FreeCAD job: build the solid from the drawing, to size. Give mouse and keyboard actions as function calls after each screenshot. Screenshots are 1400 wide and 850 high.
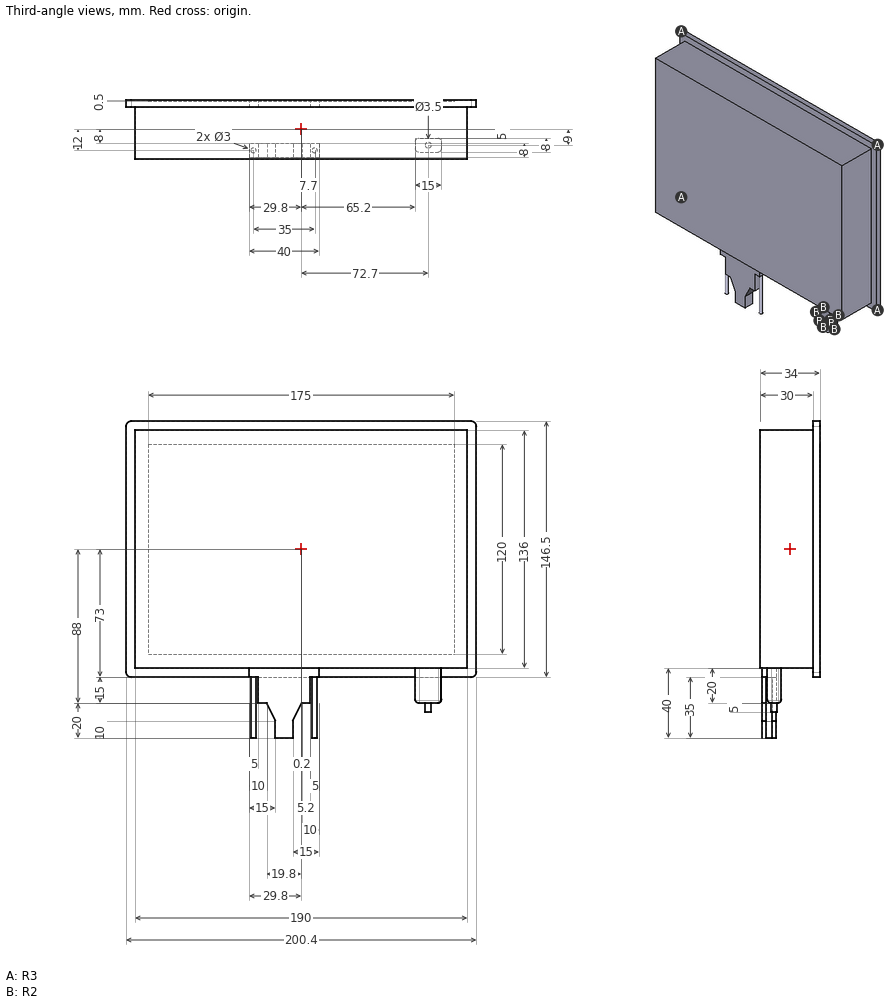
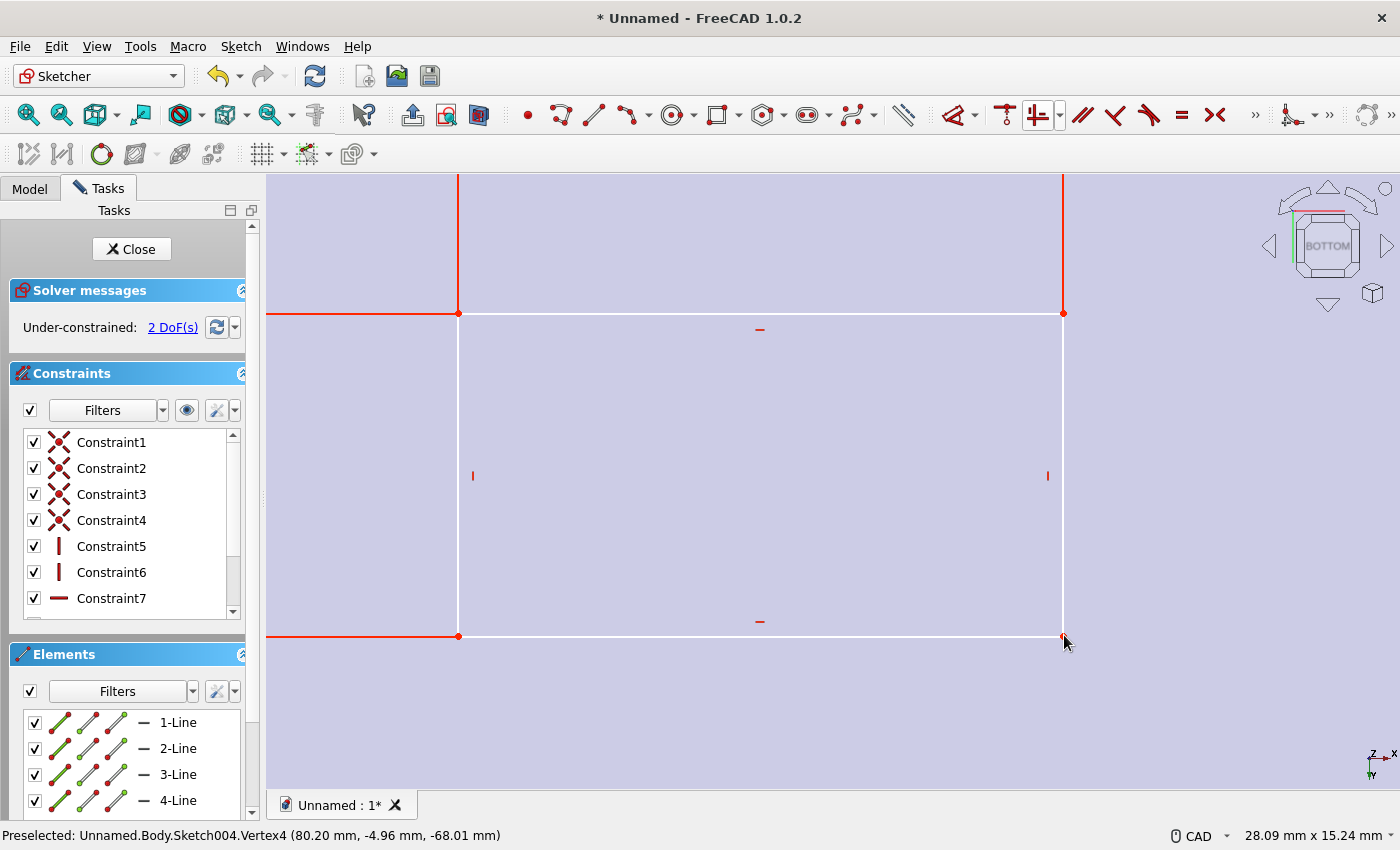
click(952, 116)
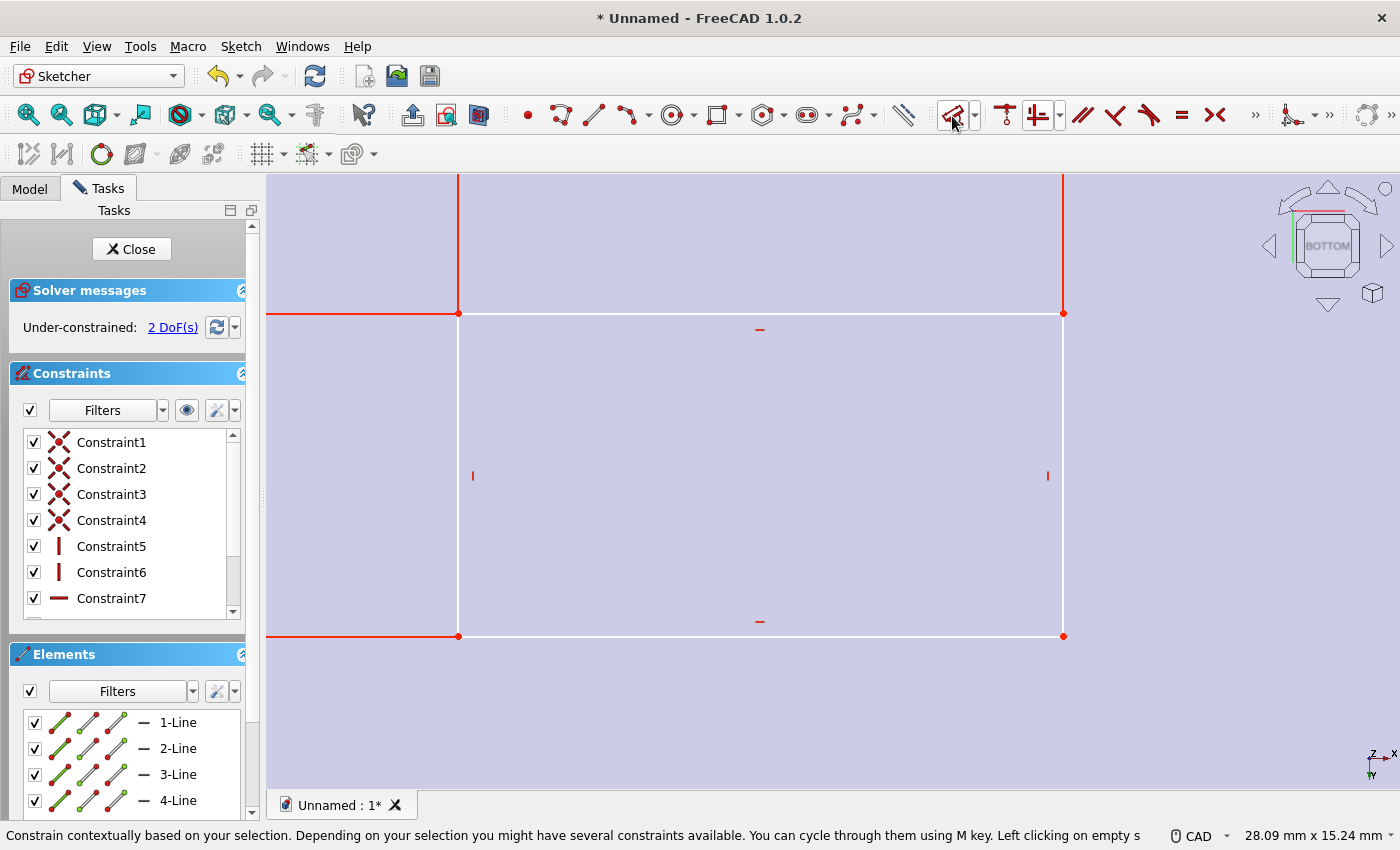
click(458, 637)
click(492, 699)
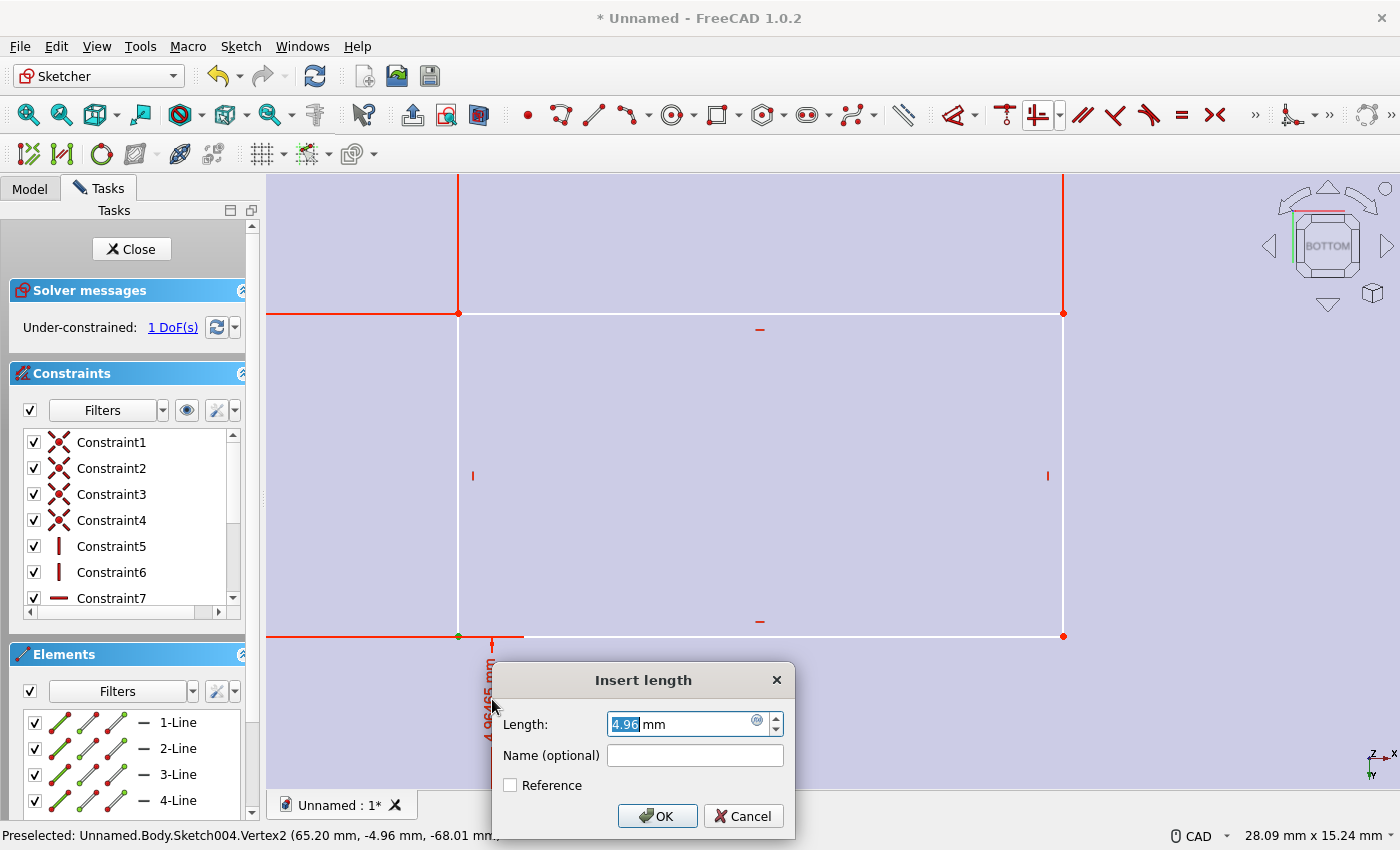
text(5)
key(Return)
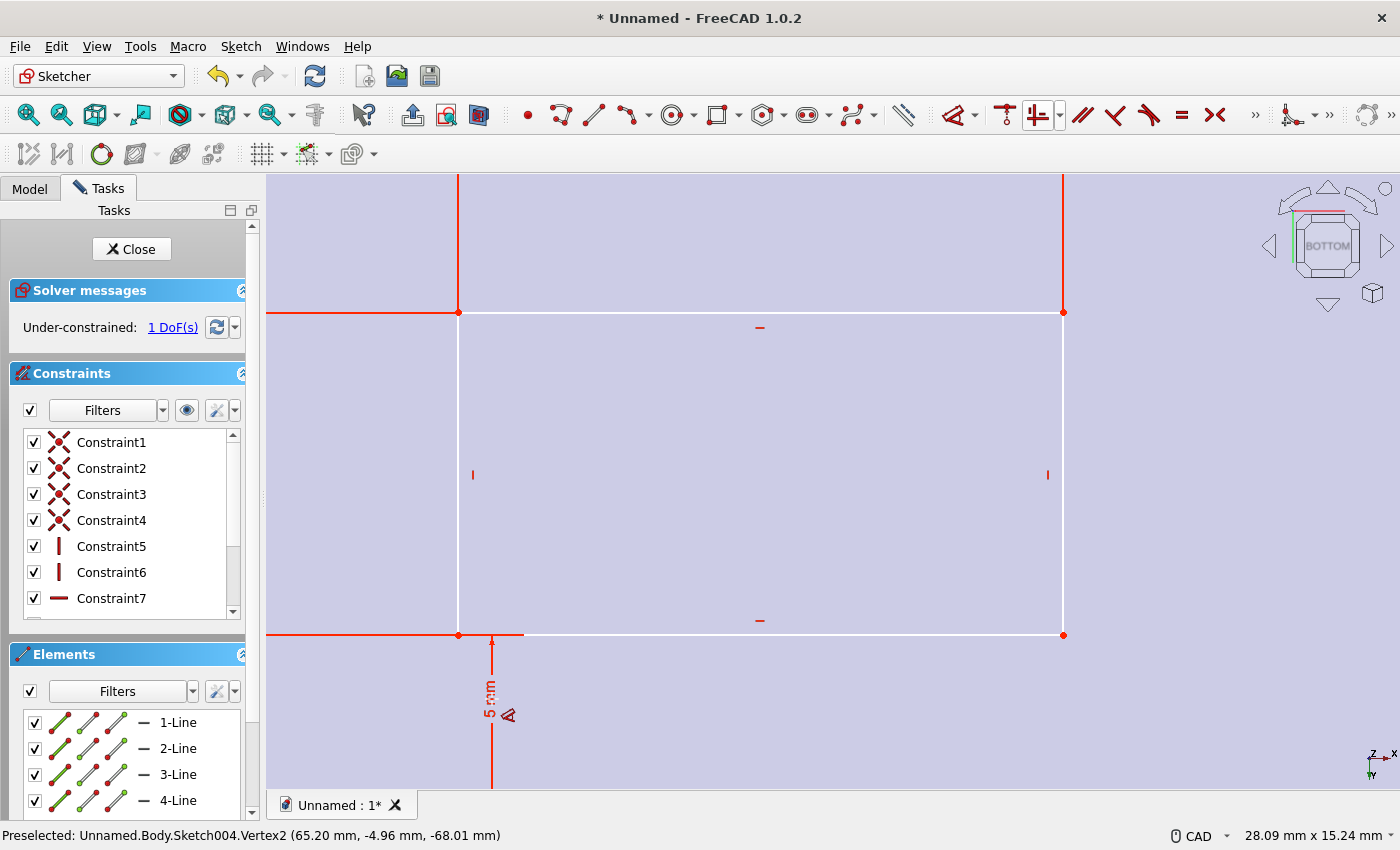
click(458, 313)
click(376, 279)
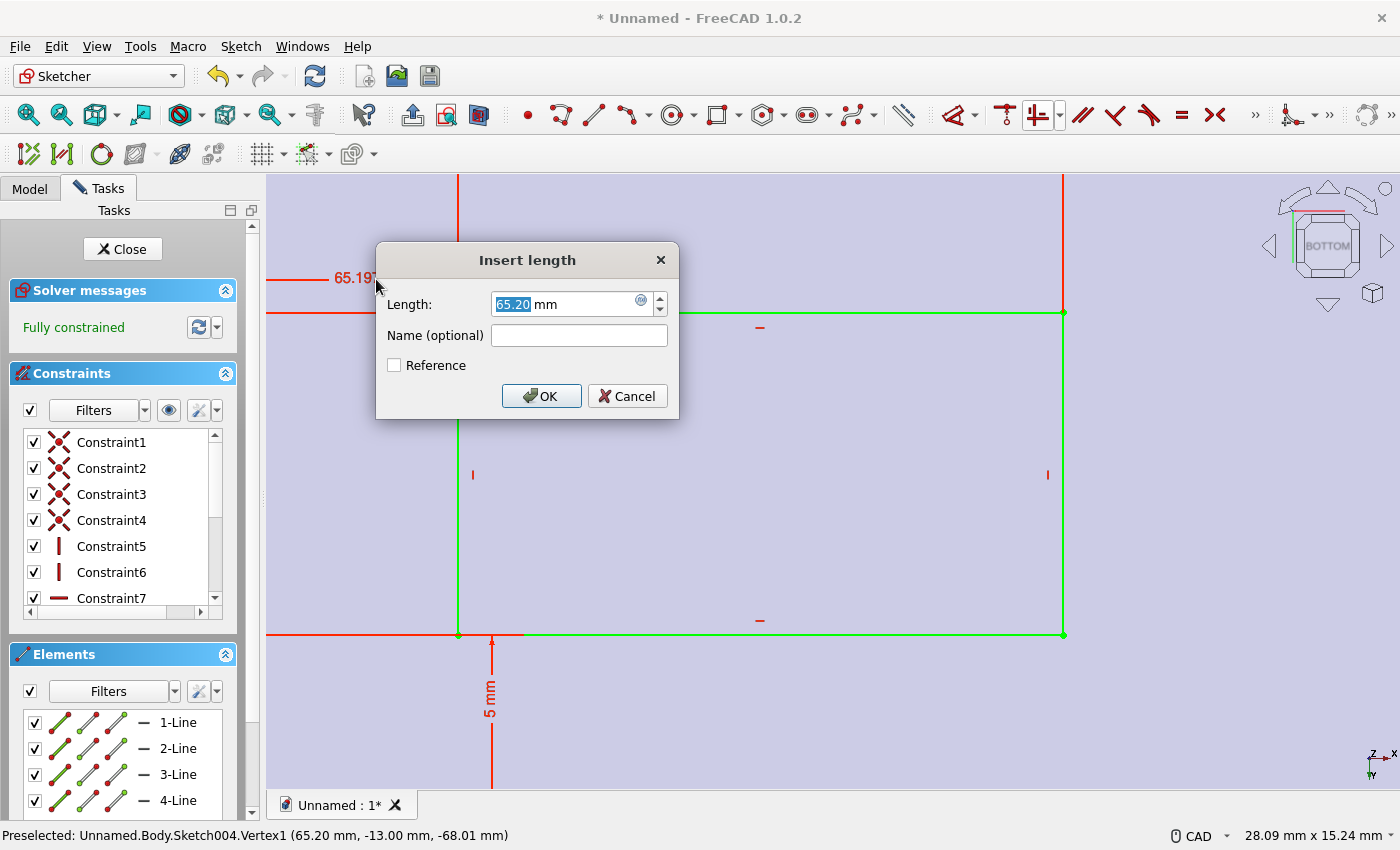
text(65.2)
key(Return)
key(Escape)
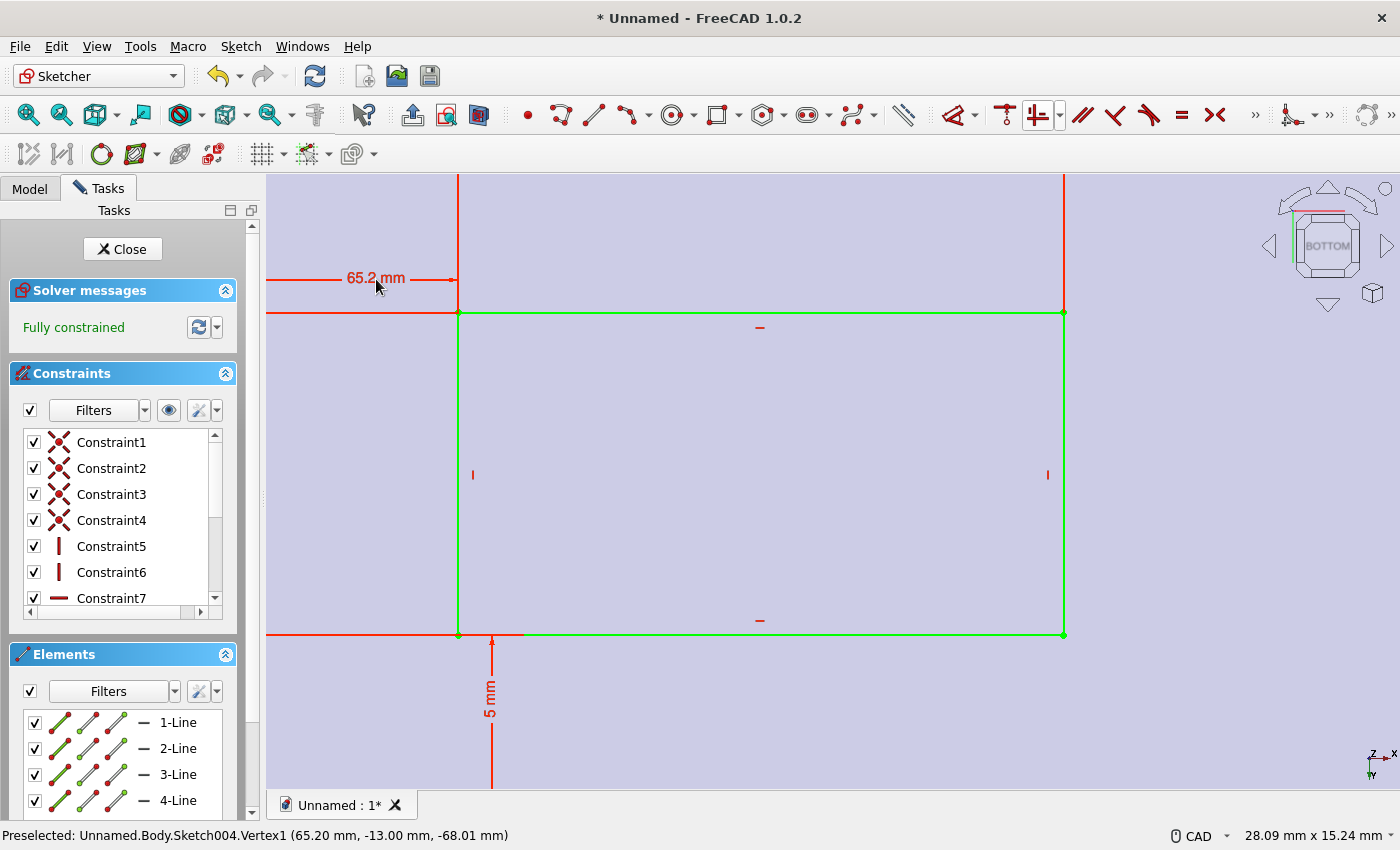
click(123, 249)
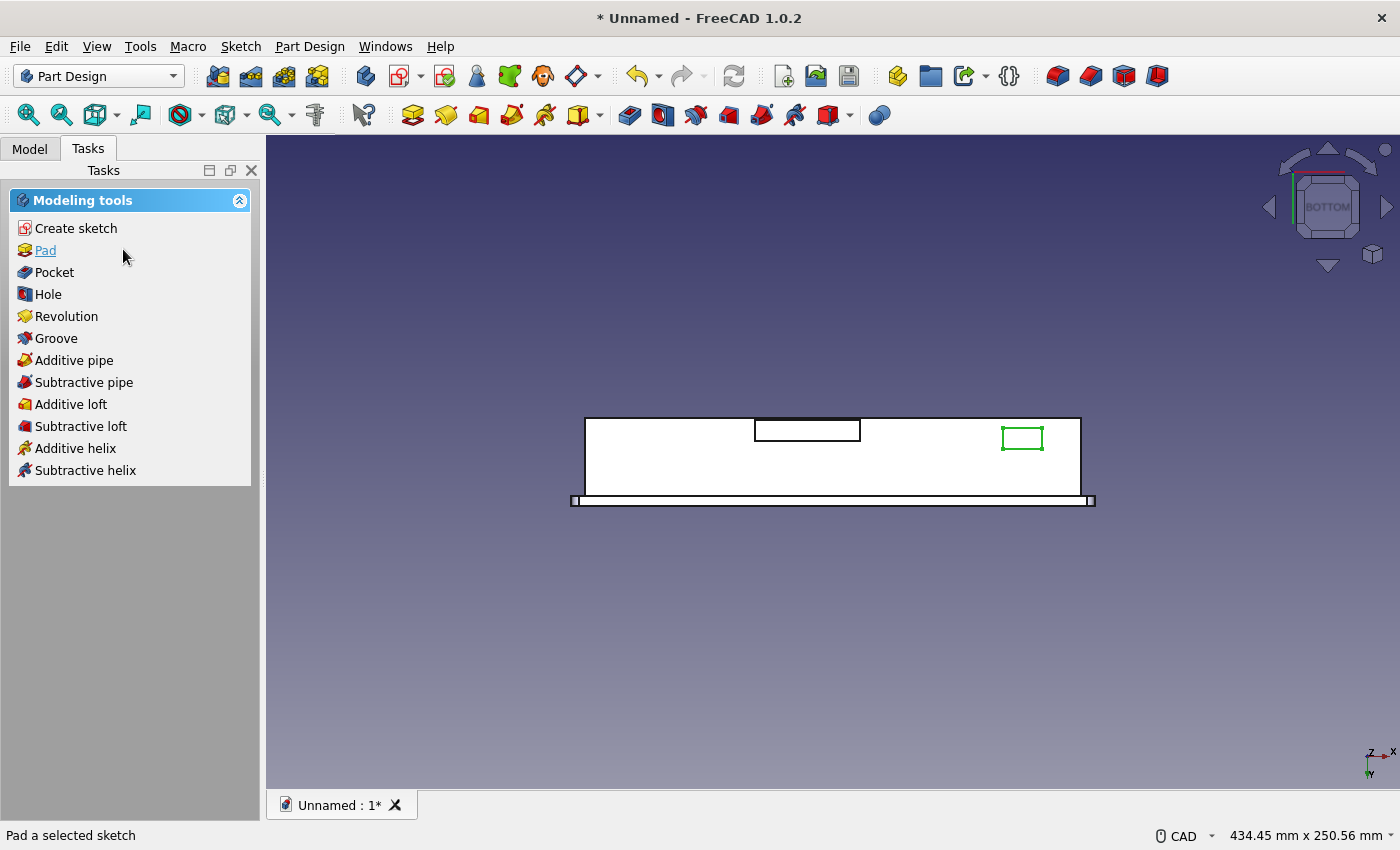
click(413, 116)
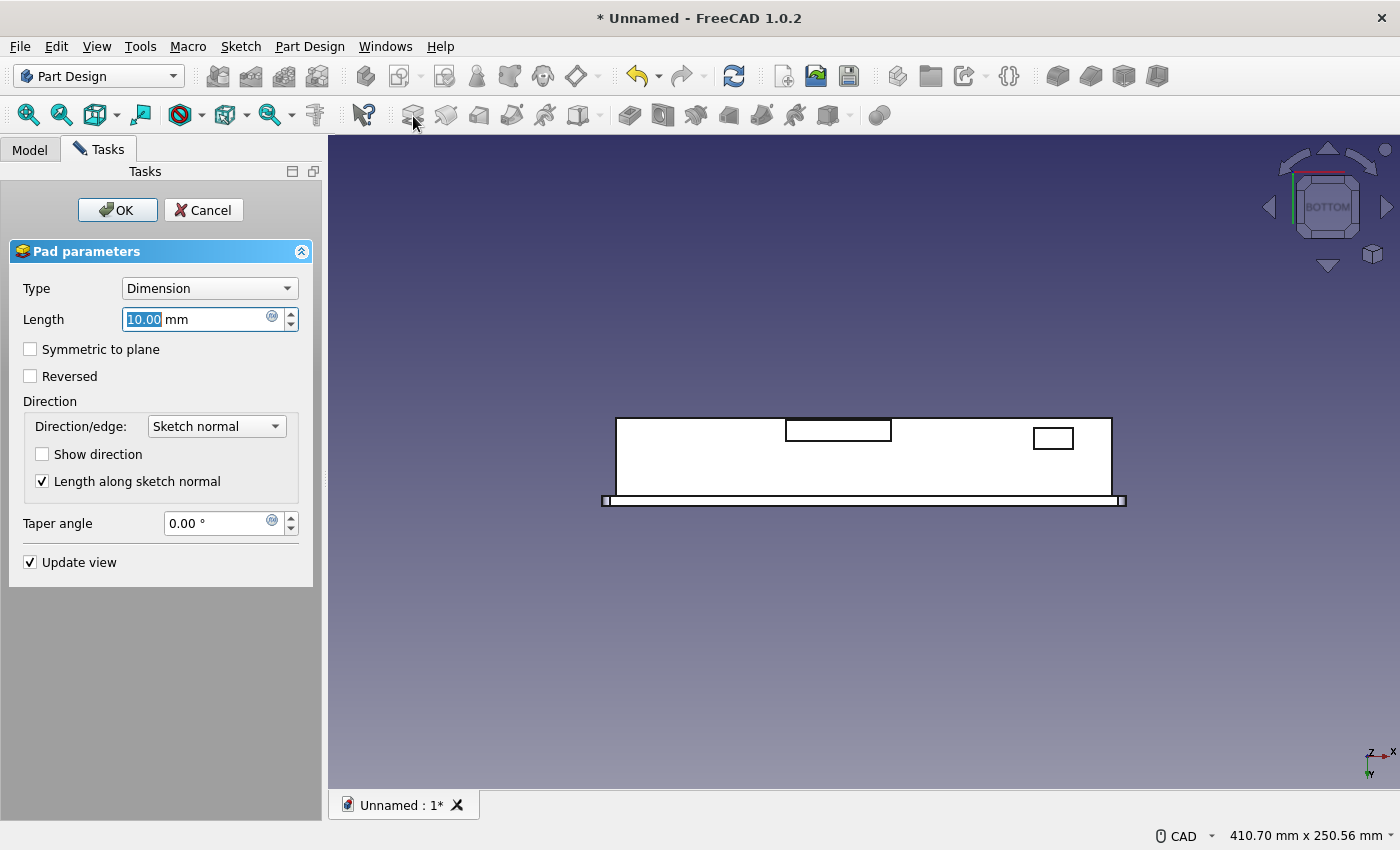
text(20)
key(Tab)